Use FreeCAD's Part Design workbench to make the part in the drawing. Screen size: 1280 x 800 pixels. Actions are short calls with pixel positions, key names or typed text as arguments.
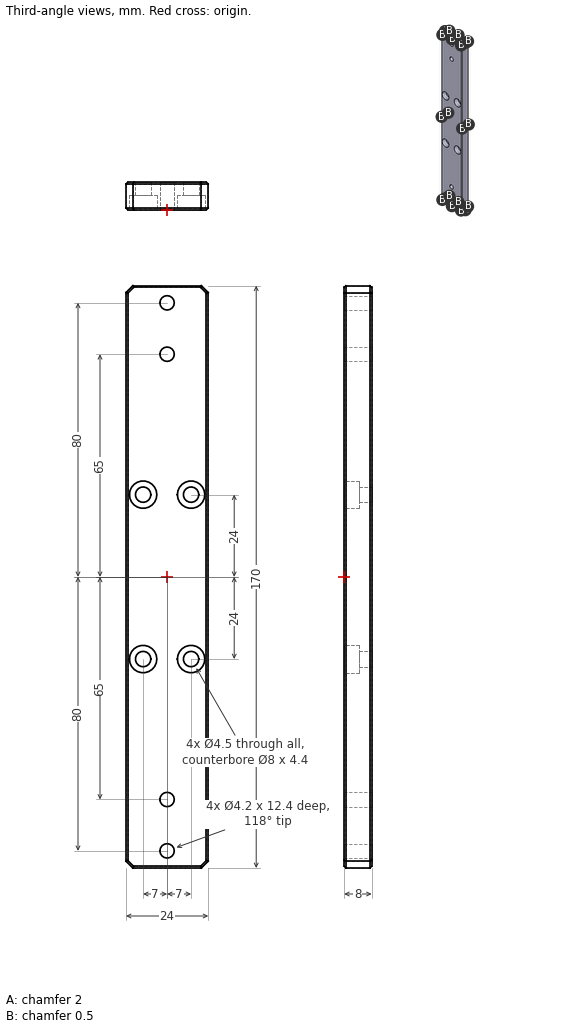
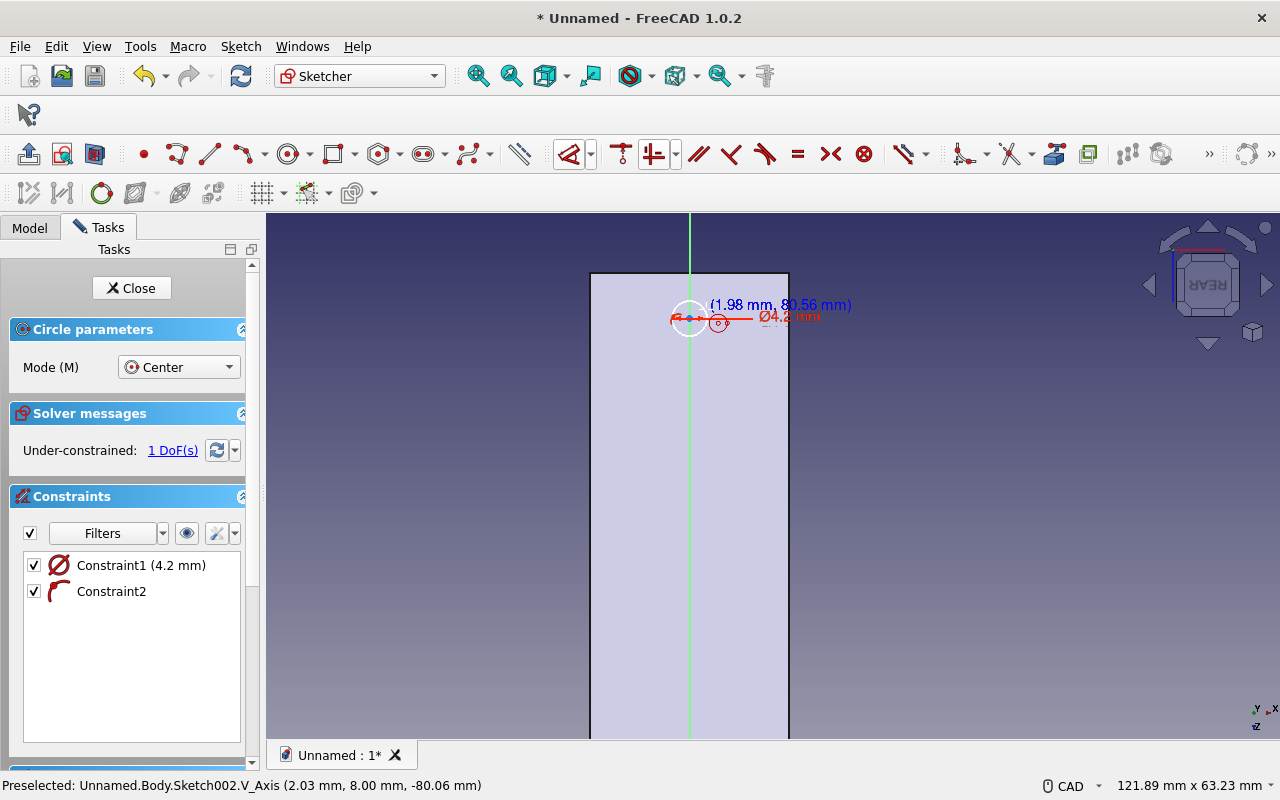
scroll(709, 311, down, 7)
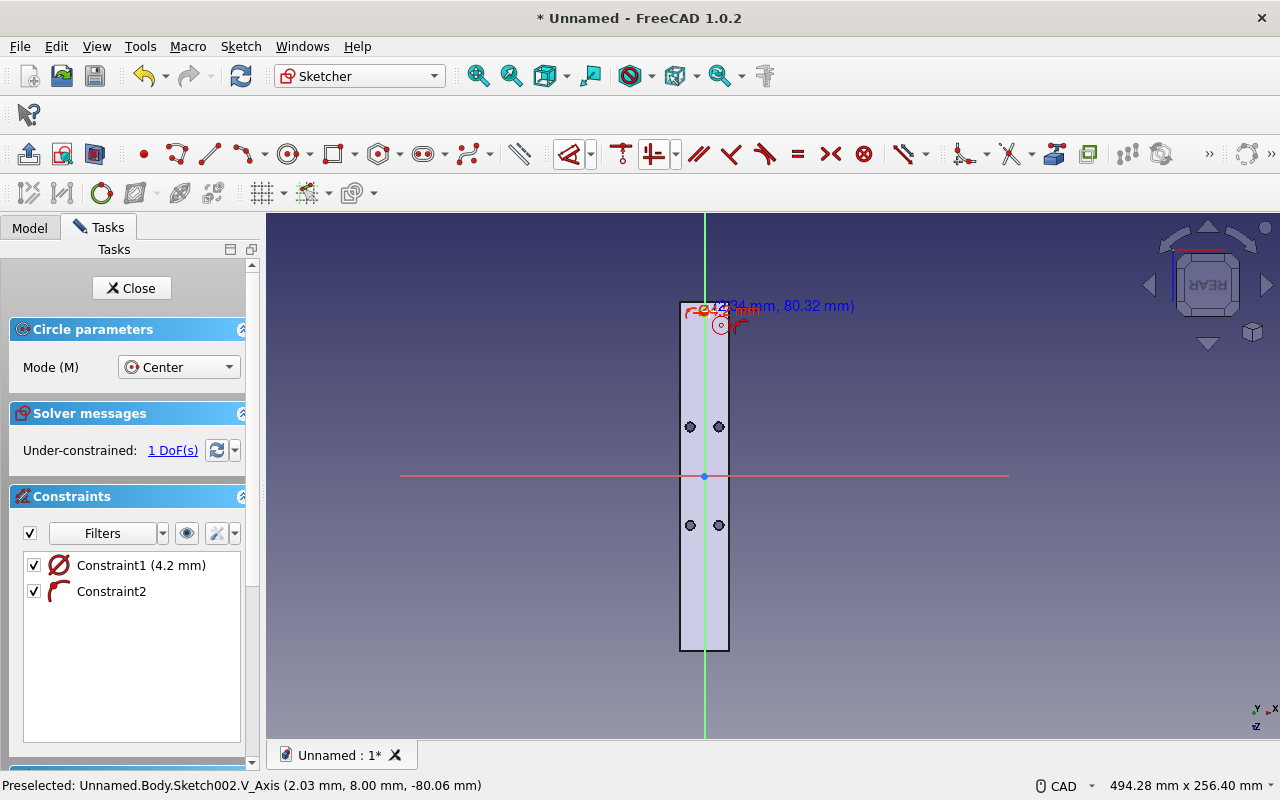
scroll(705, 640, up, 9)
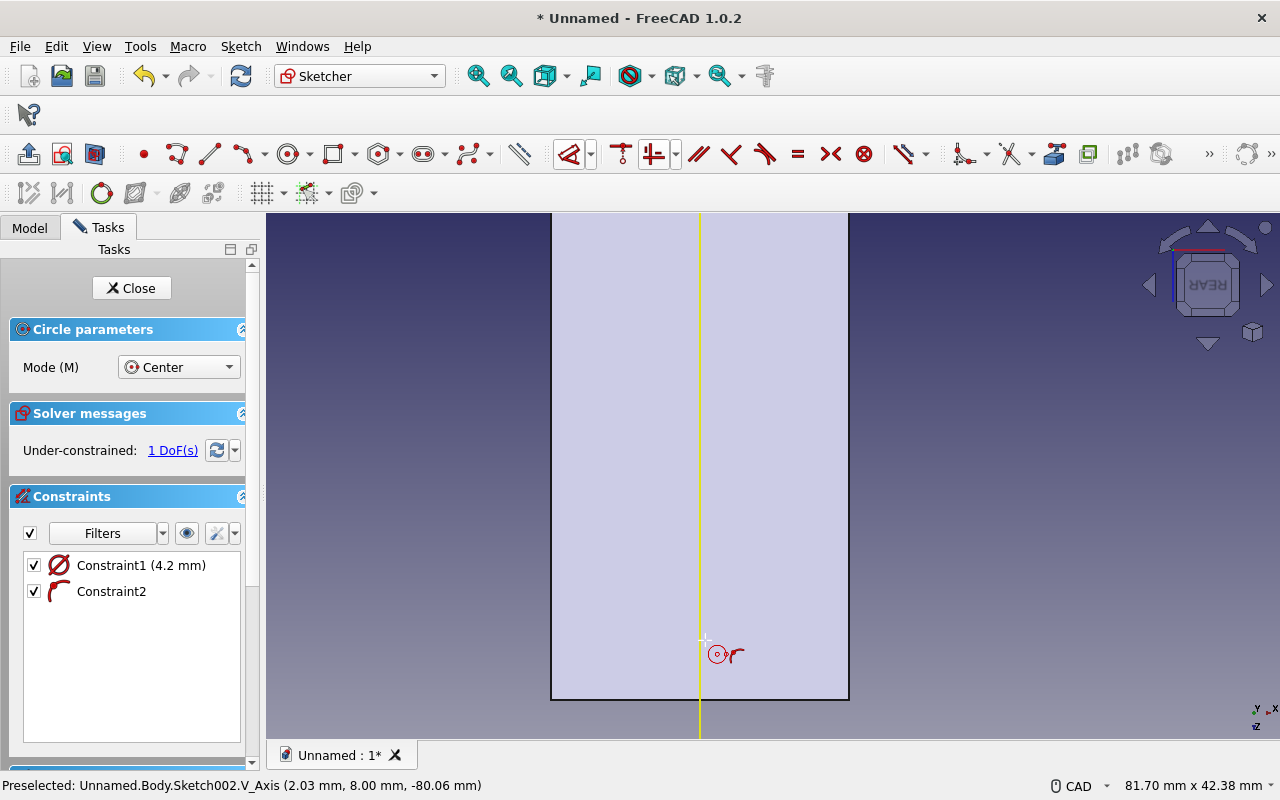
scroll(705, 641, down, 9)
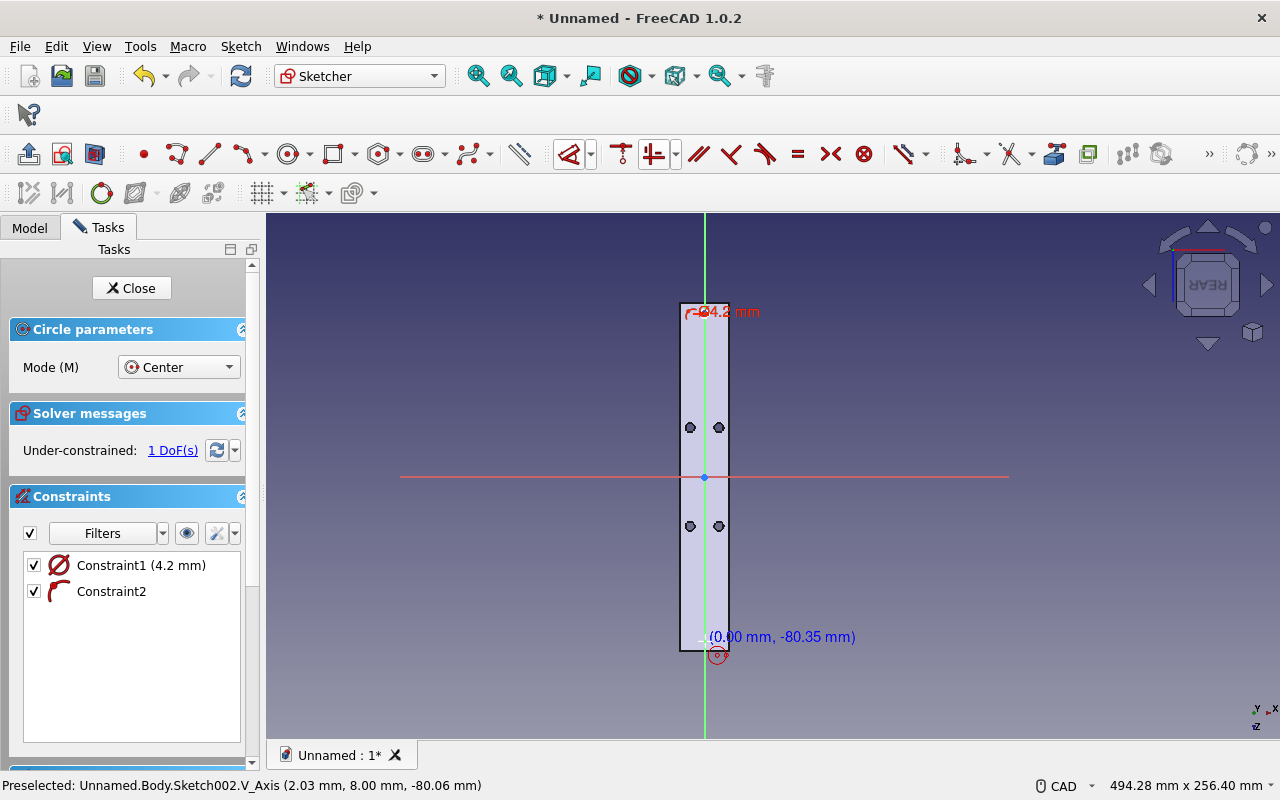
click(705, 641)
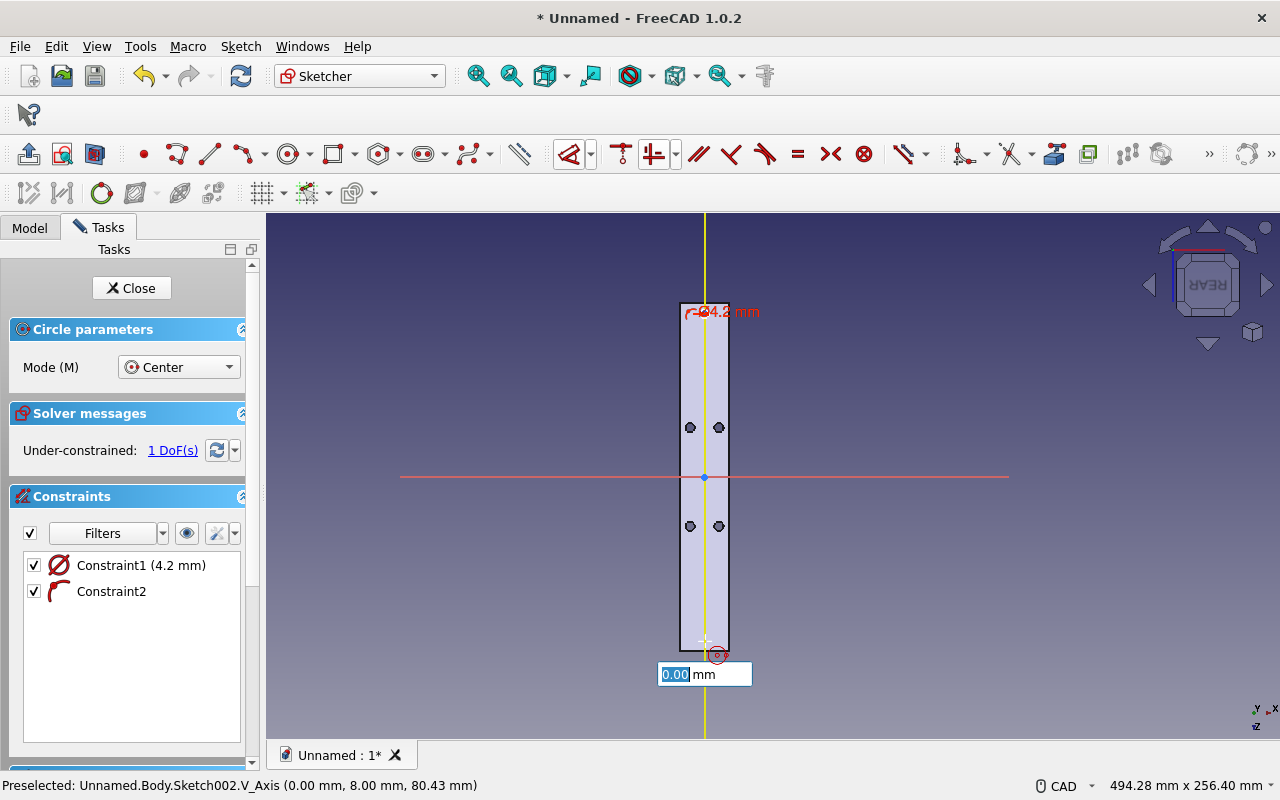
scroll(709, 640, up, 7)
move(706, 636)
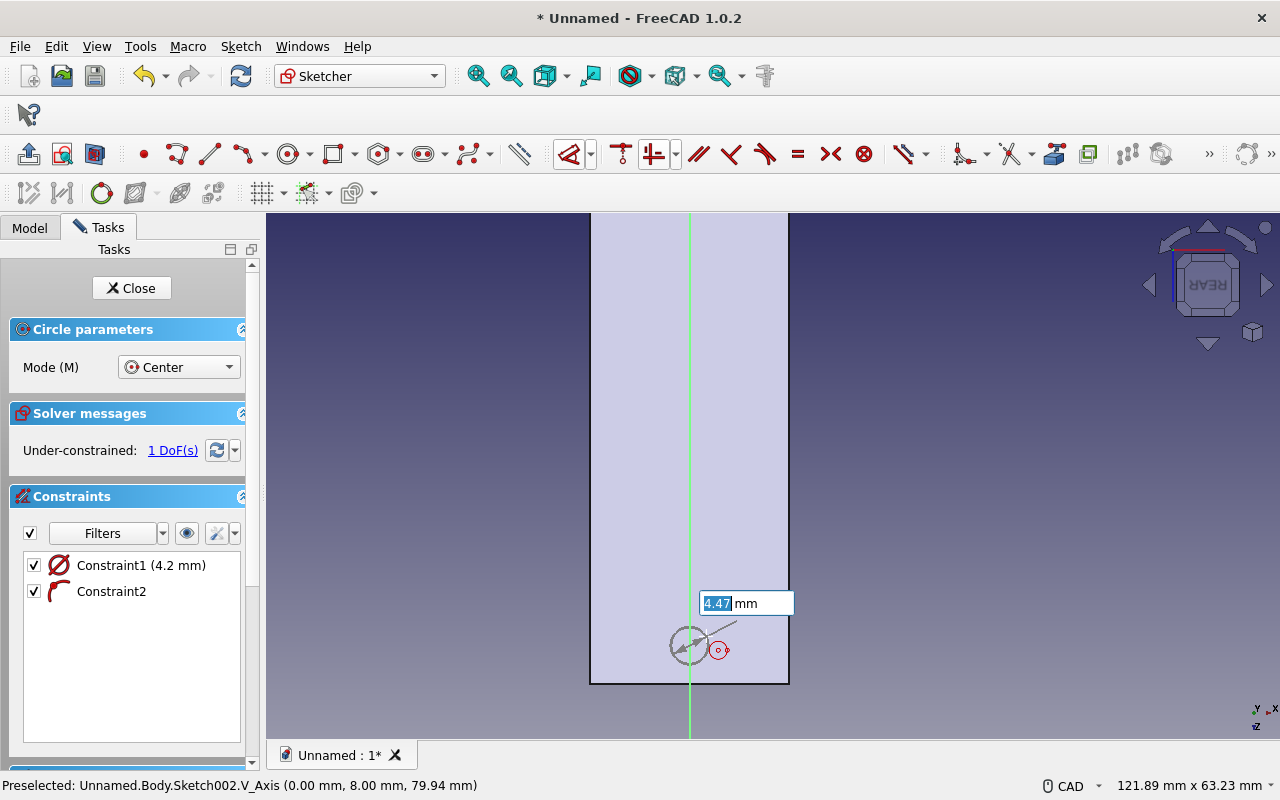
text(4.2)
key(Return)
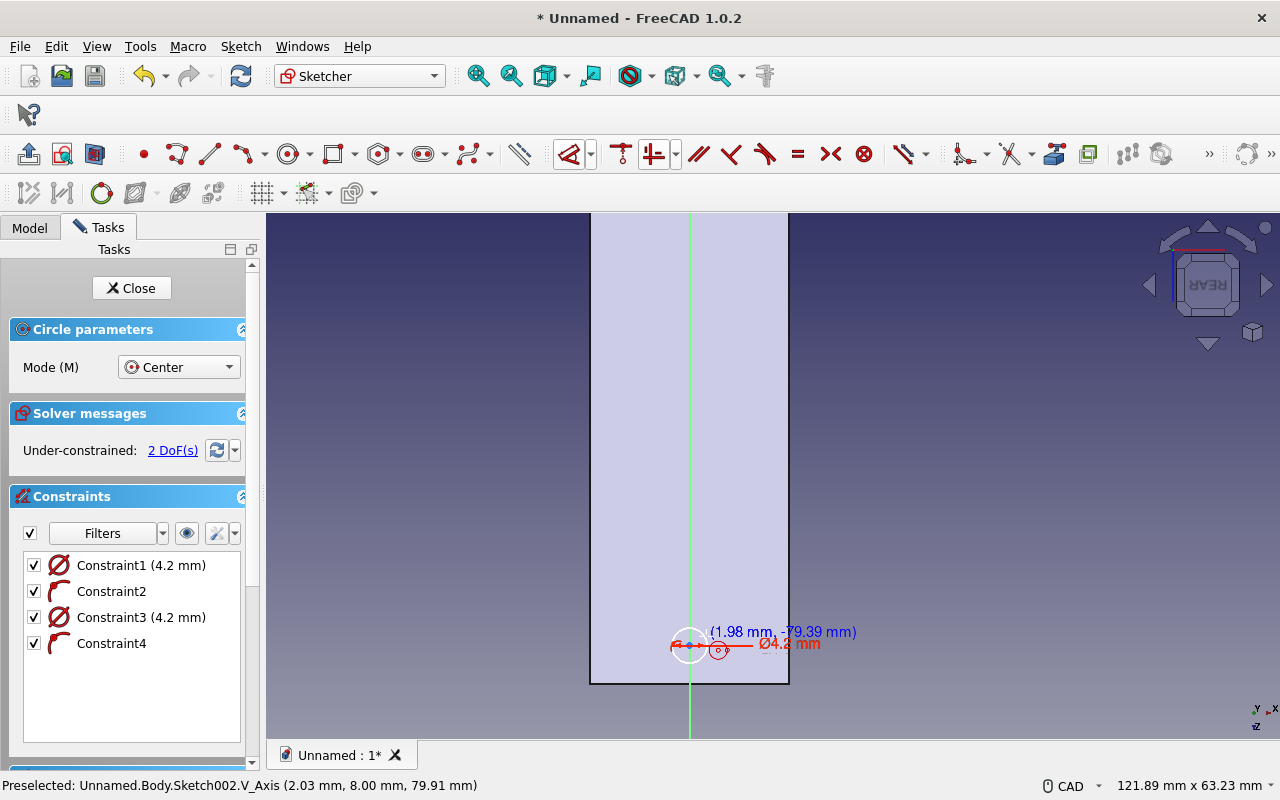
scroll(690, 517, up, 2)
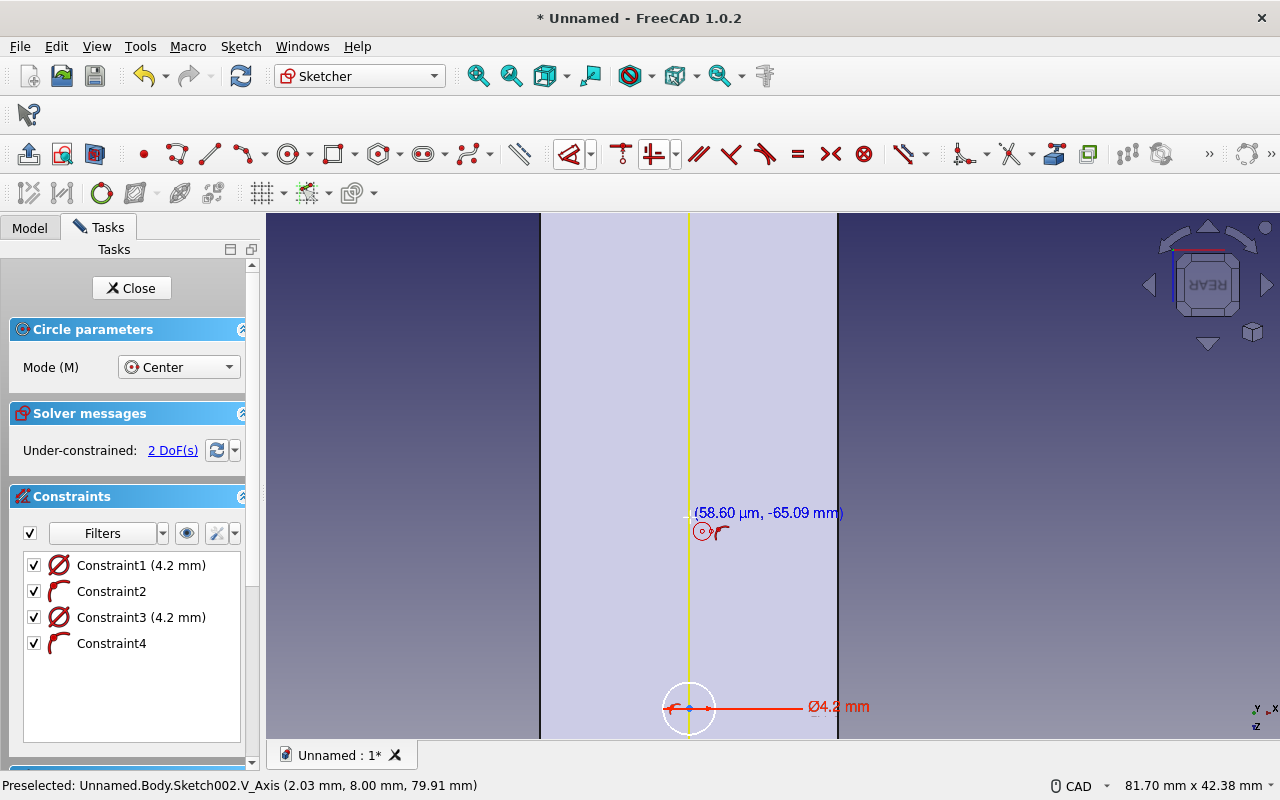
scroll(708, 628, down, 9)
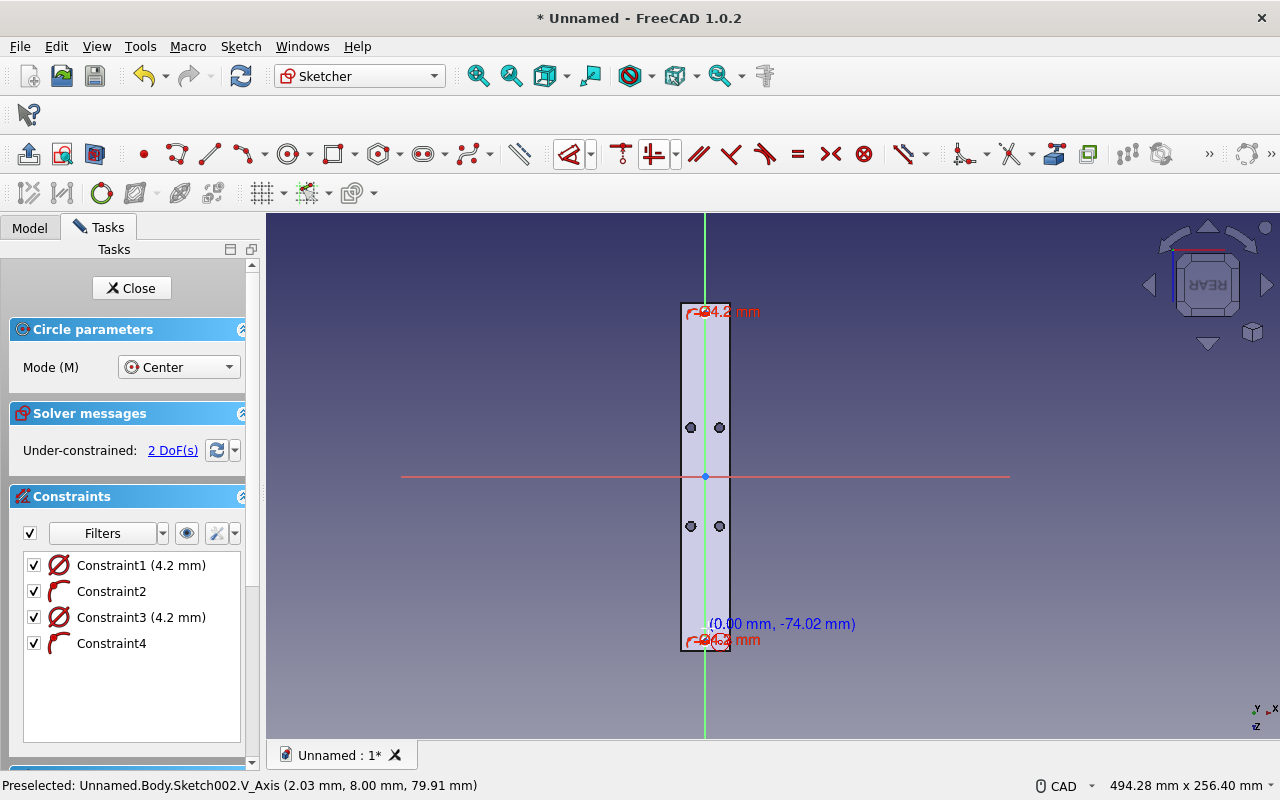
click(705, 610)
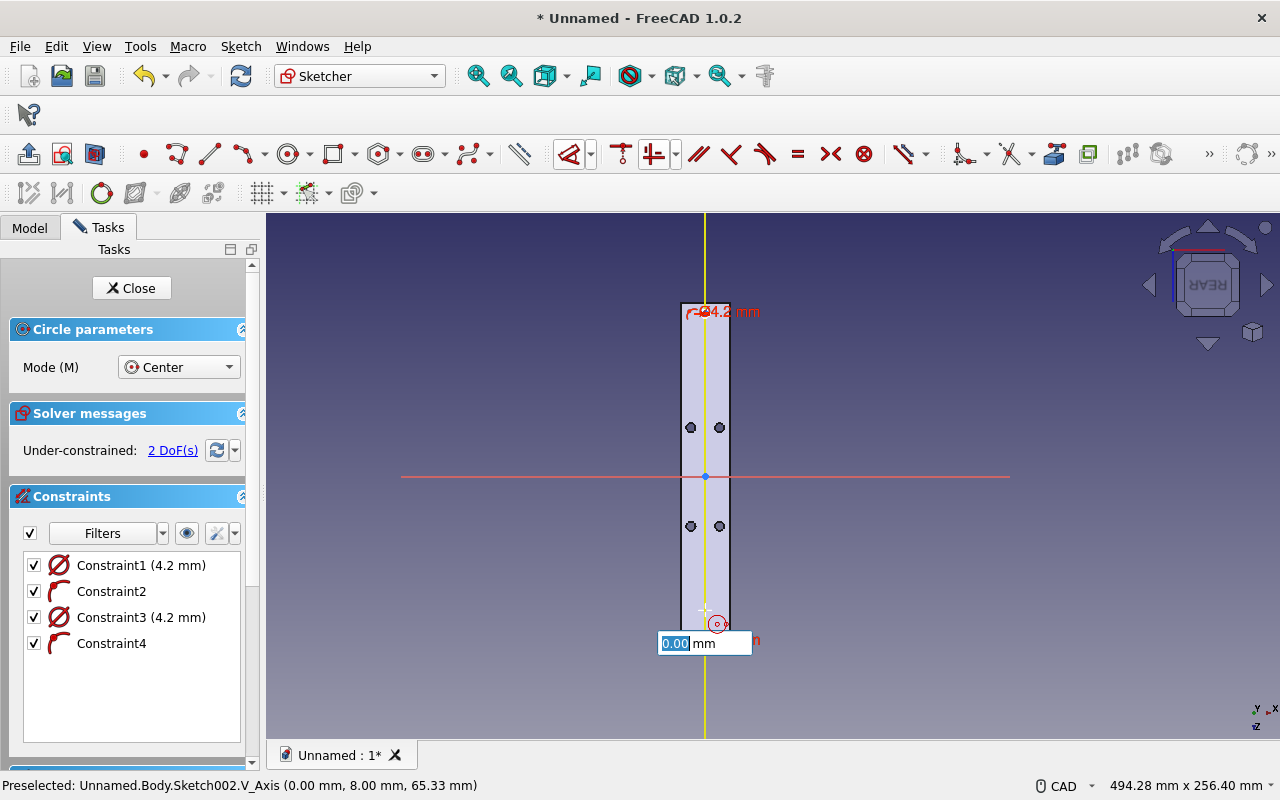
scroll(709, 609, up, 7)
move(709, 606)